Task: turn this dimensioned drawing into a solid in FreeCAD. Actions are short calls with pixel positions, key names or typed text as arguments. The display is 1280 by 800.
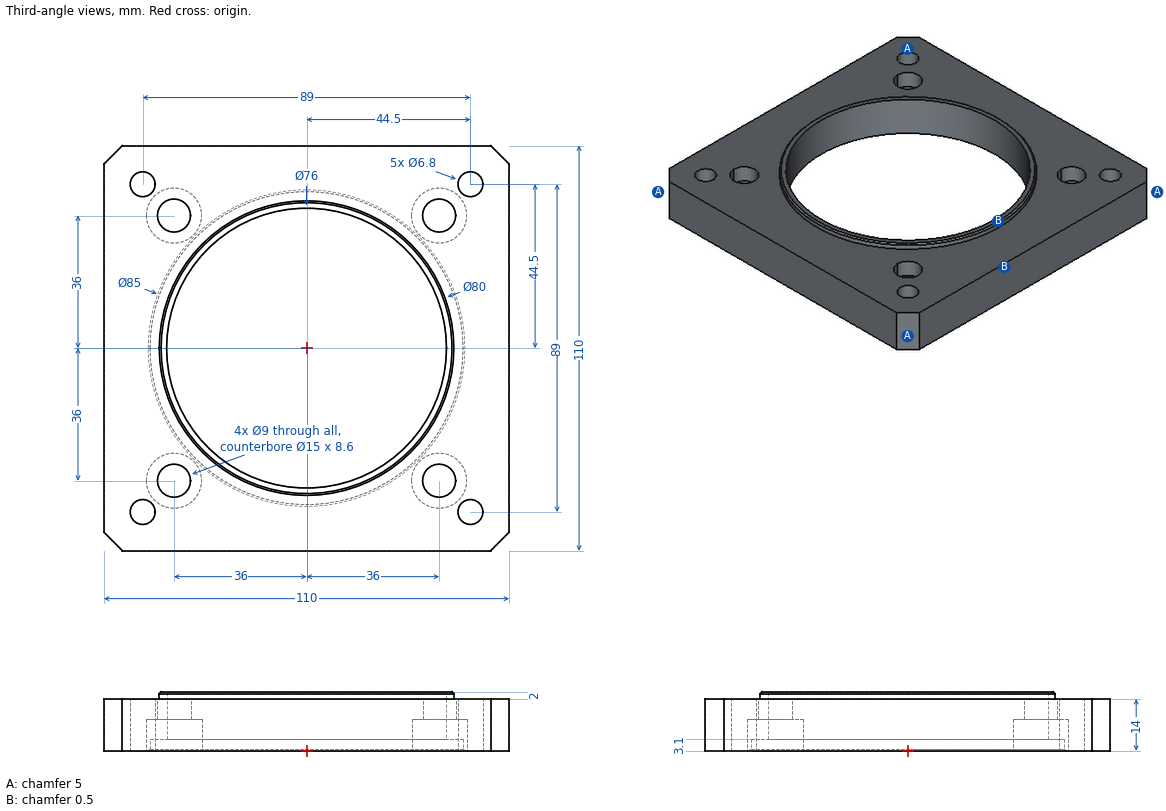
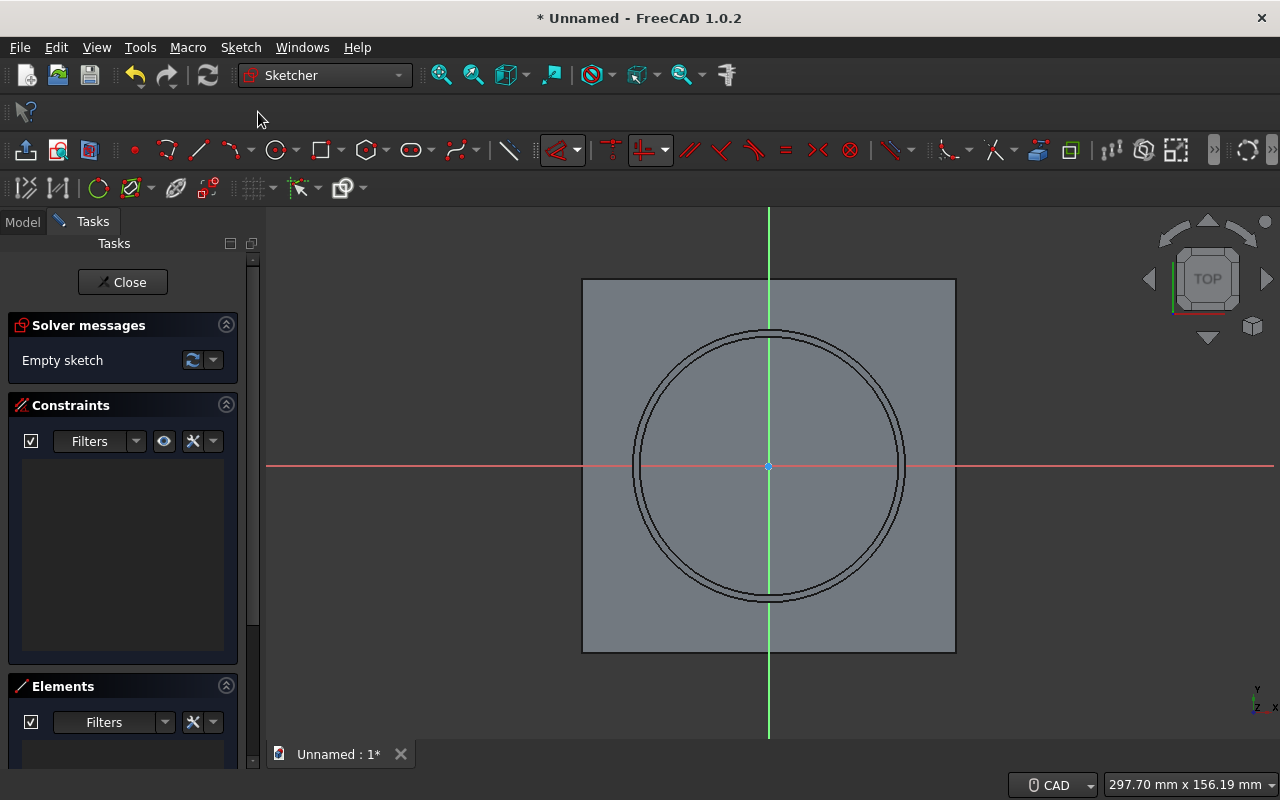
click(90, 150)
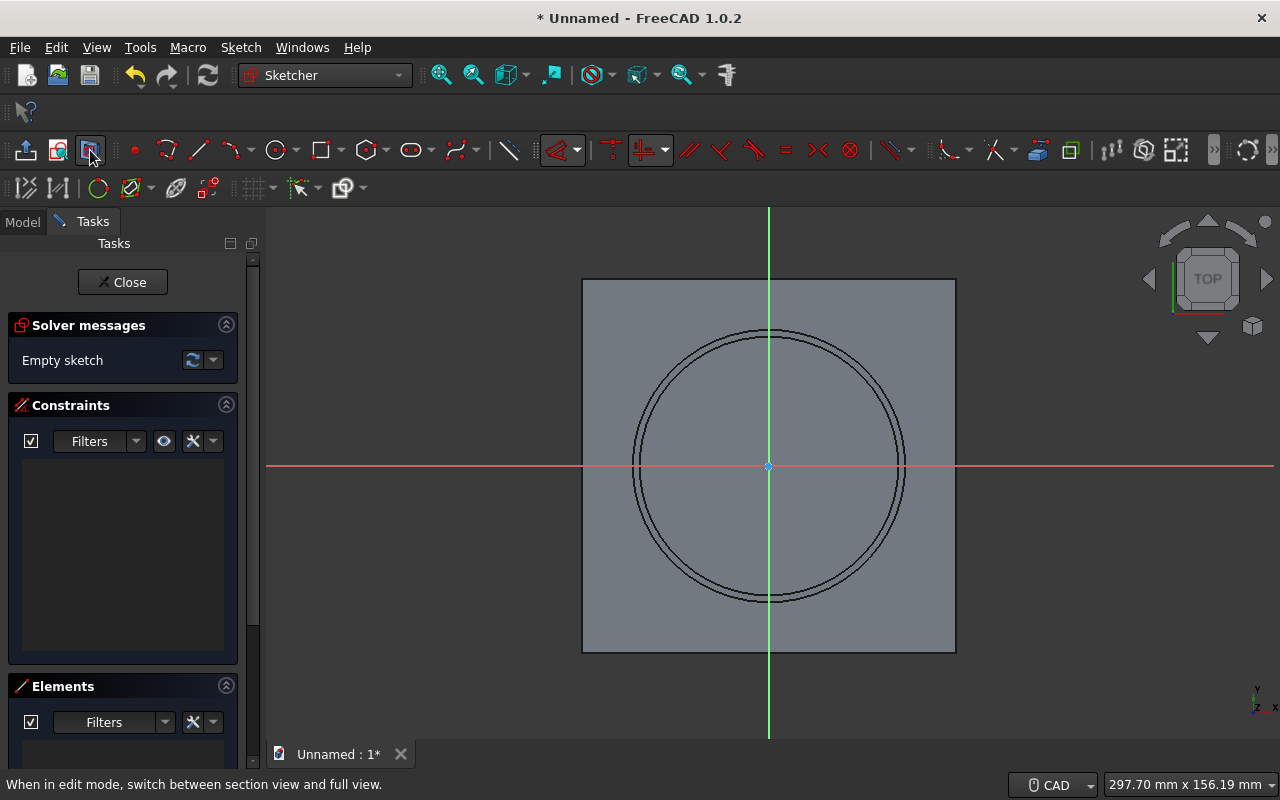
click(276, 150)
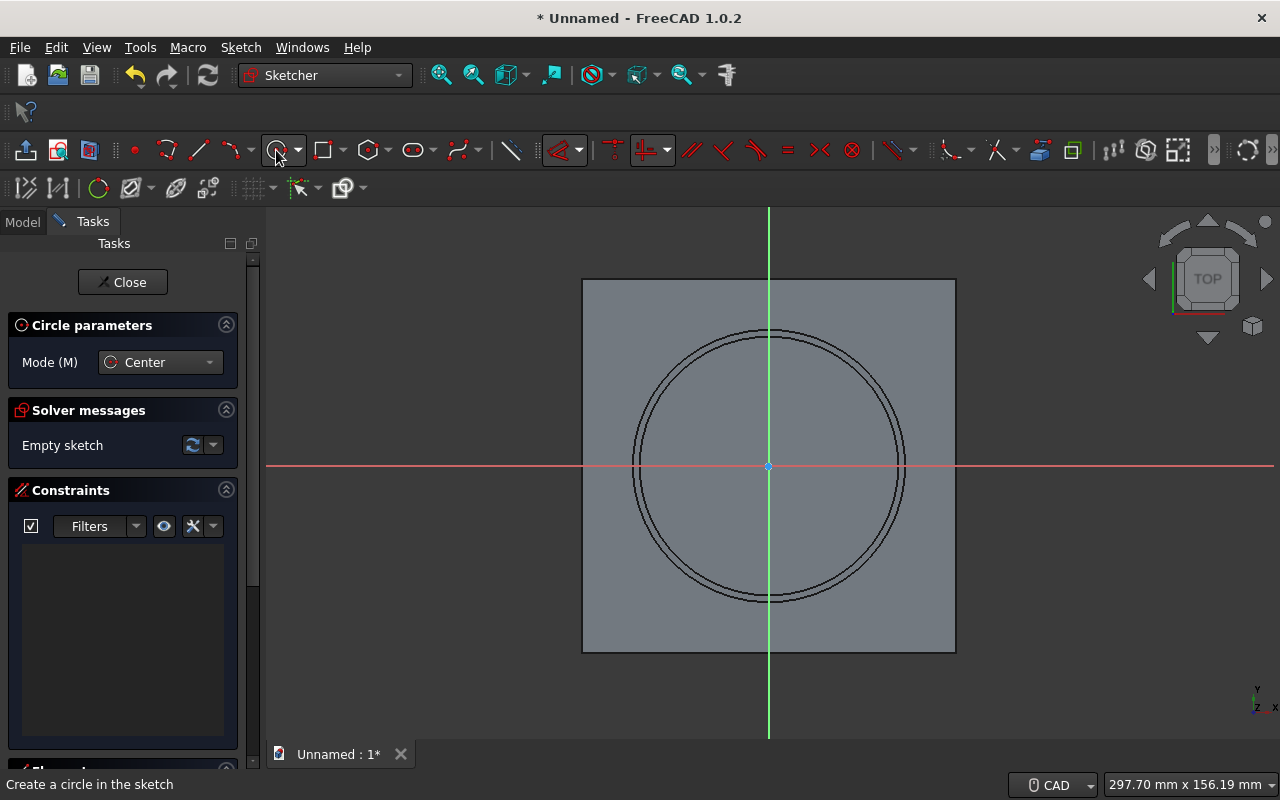
click(769, 466)
click(861, 375)
key(Escape)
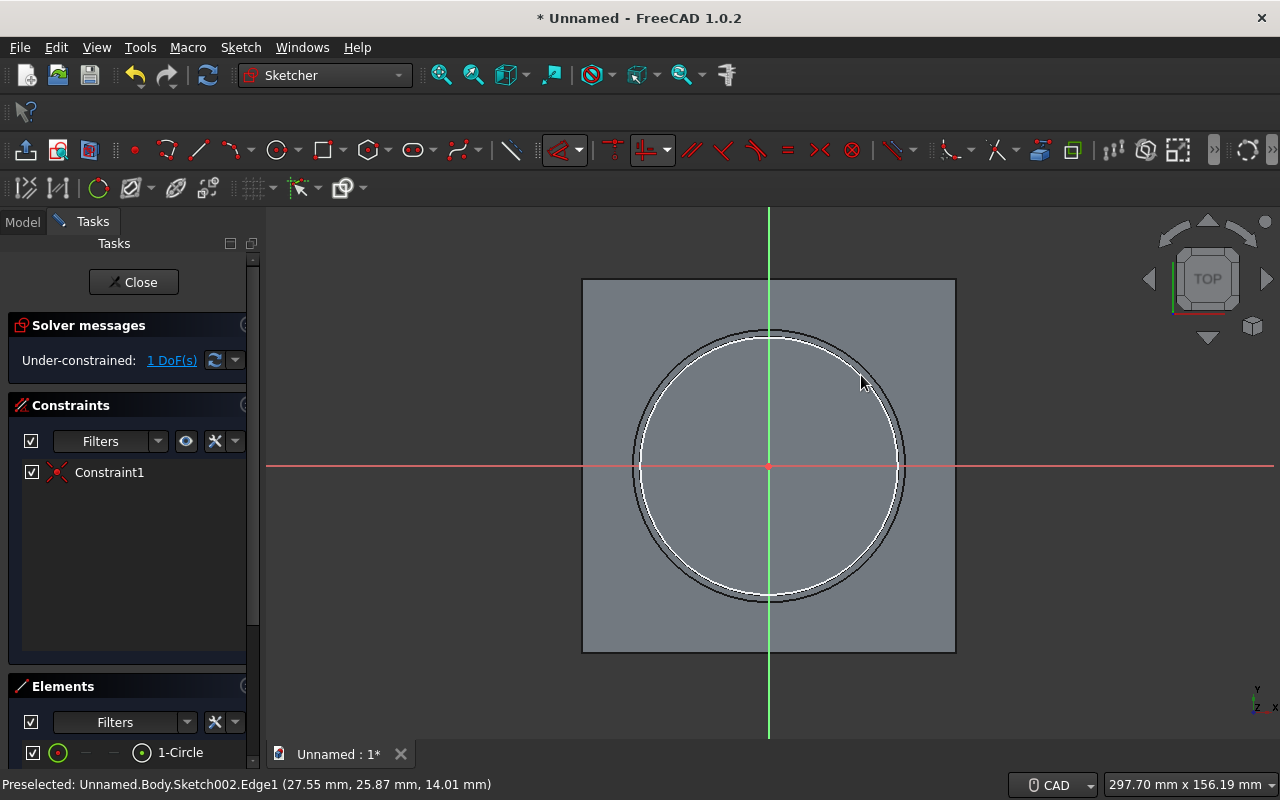
click(860, 375)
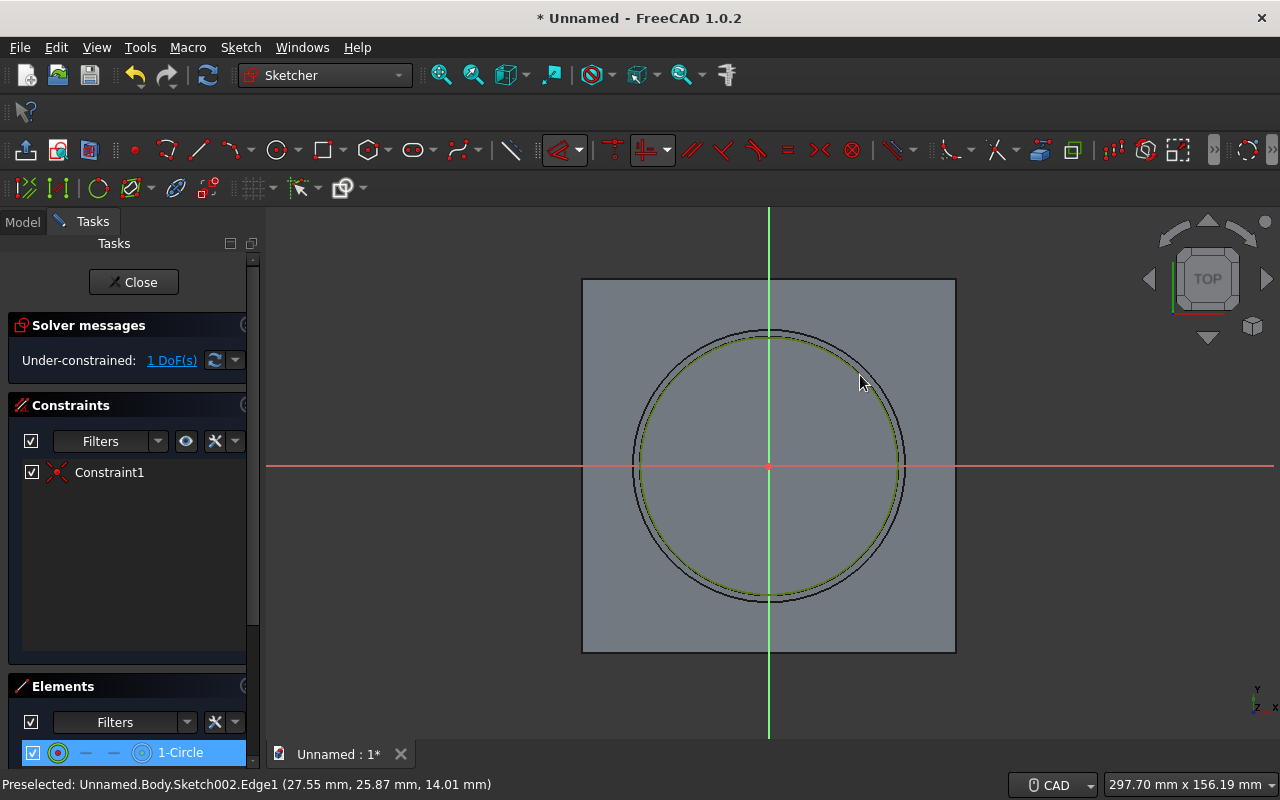
click(582, 150)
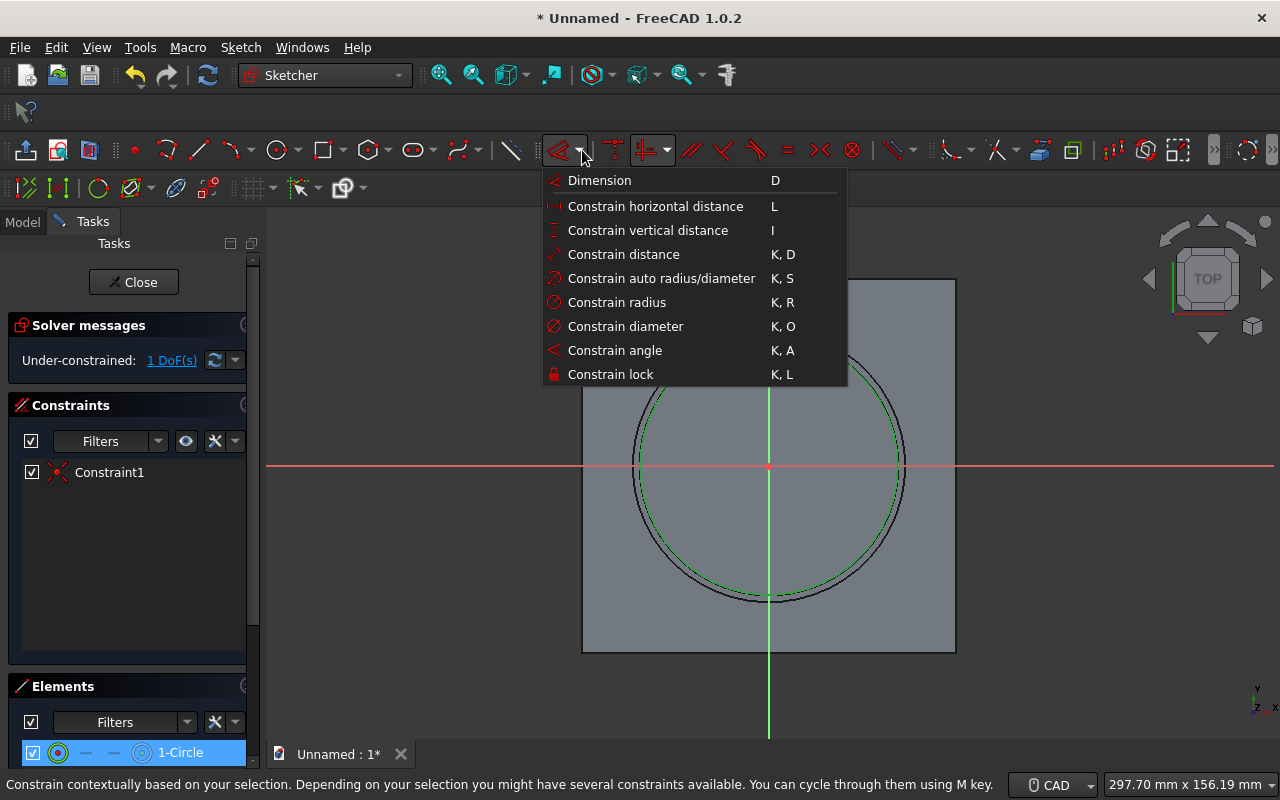
click(695, 326)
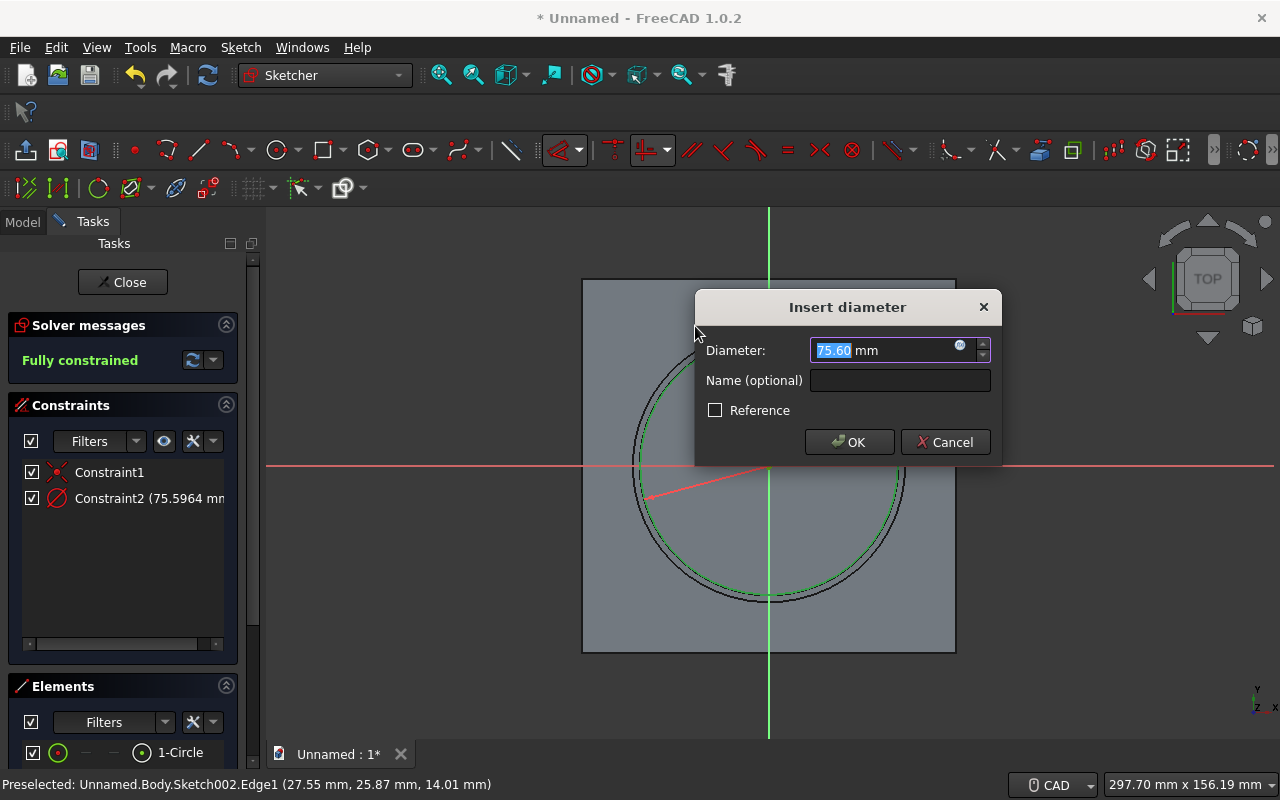
text(76)
key(Return)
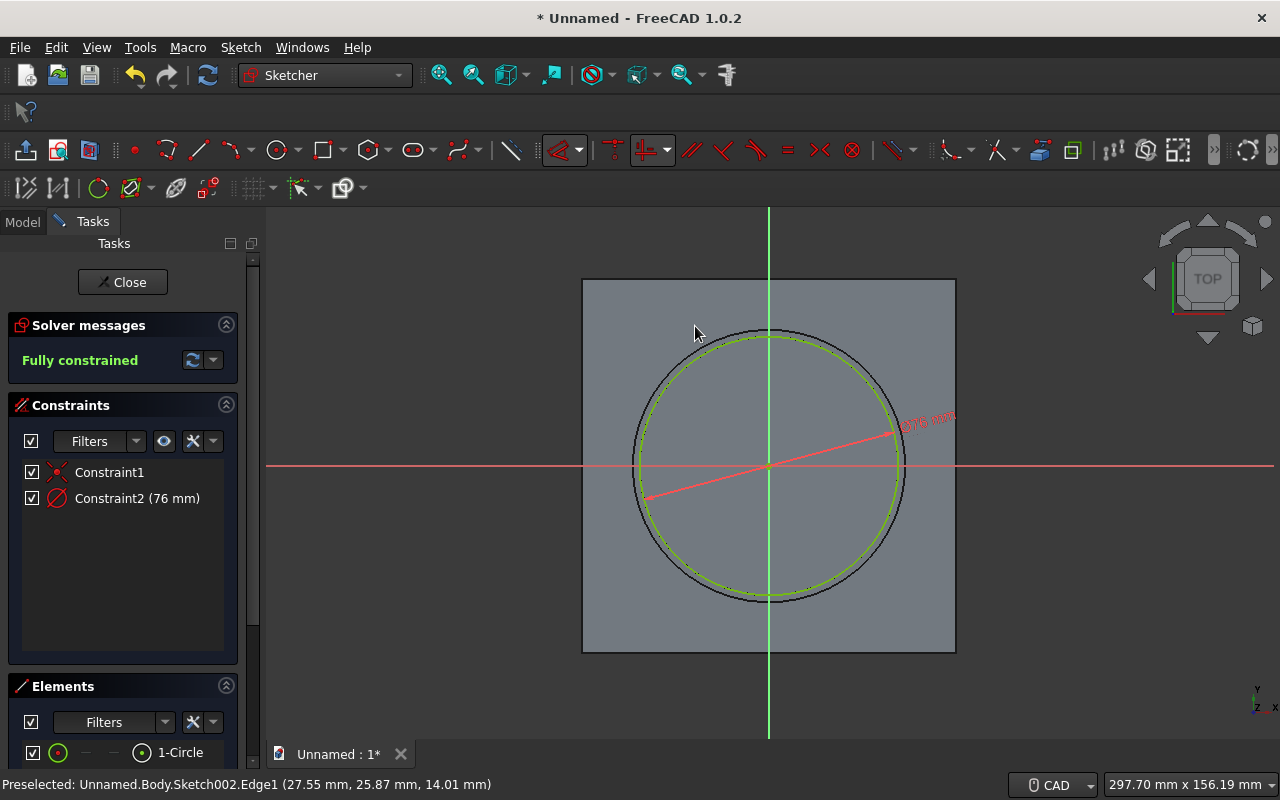
click(123, 282)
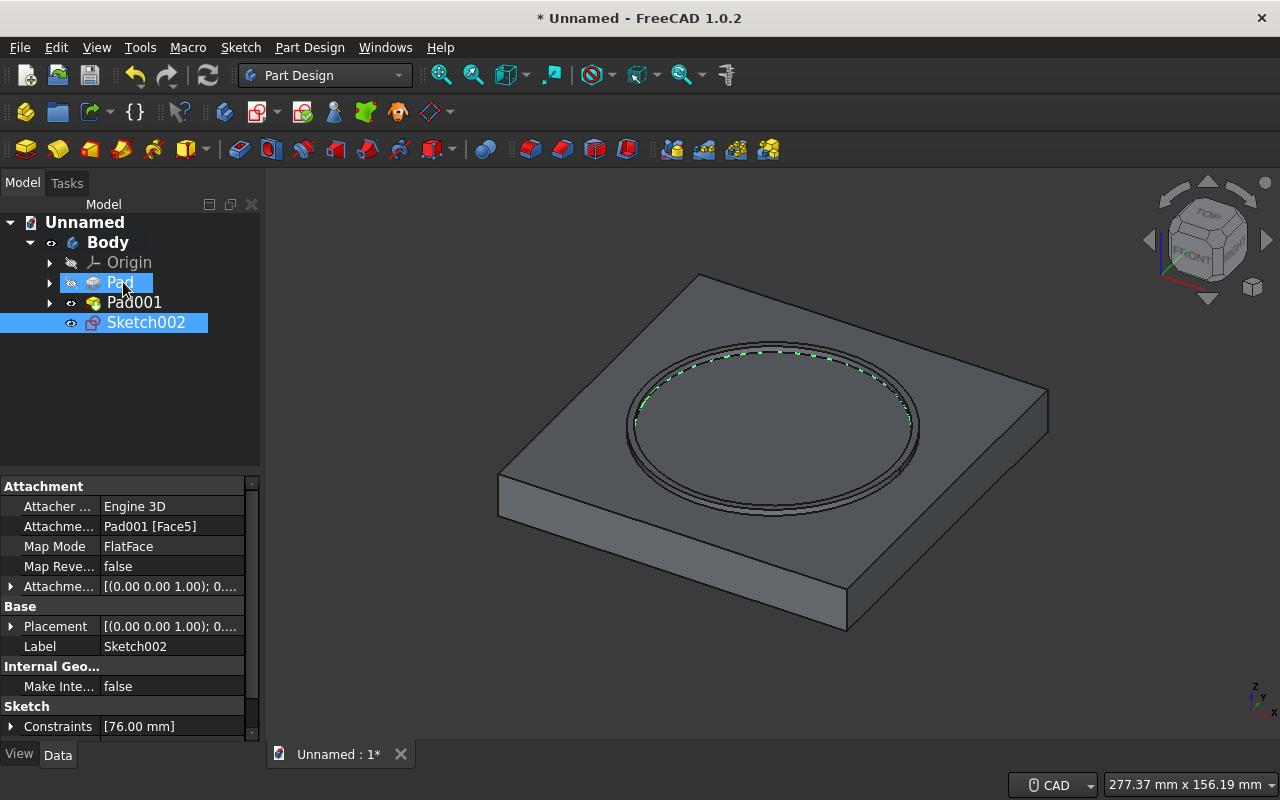
click(240, 150)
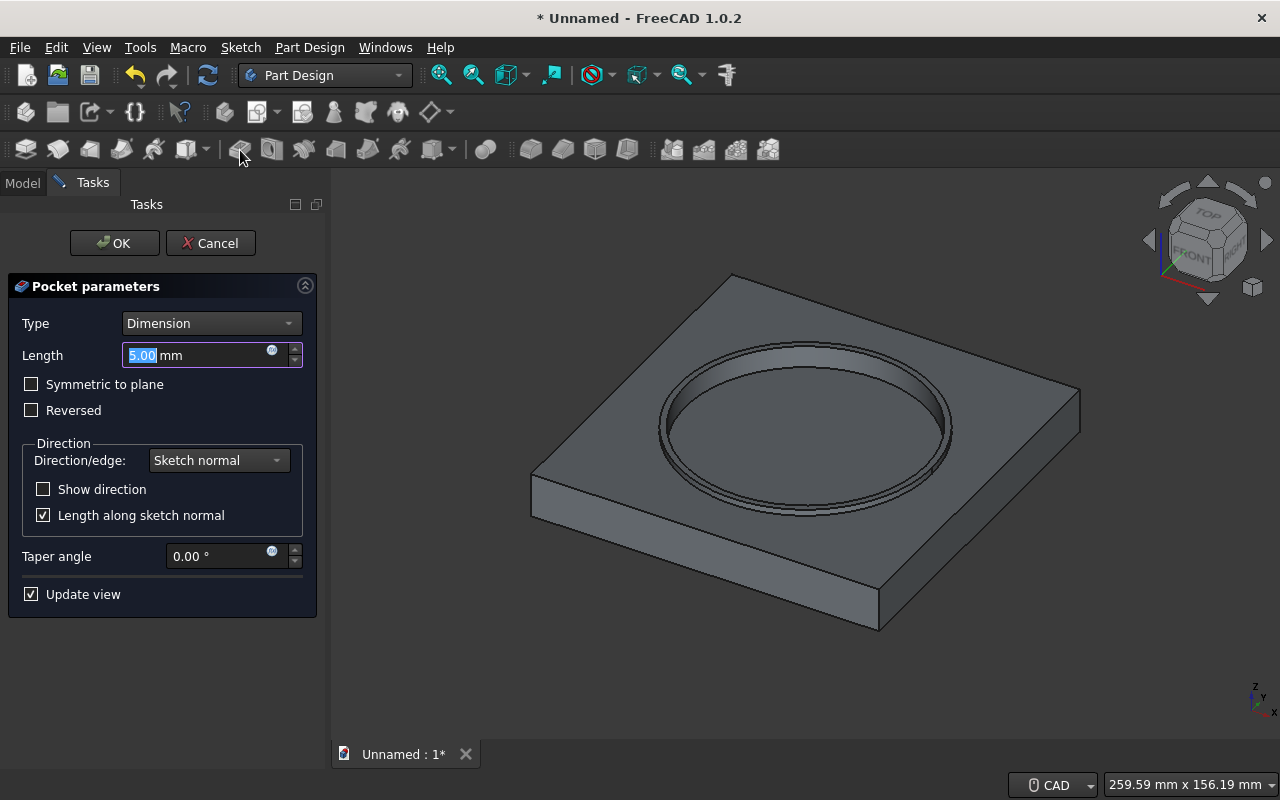
click(212, 324)